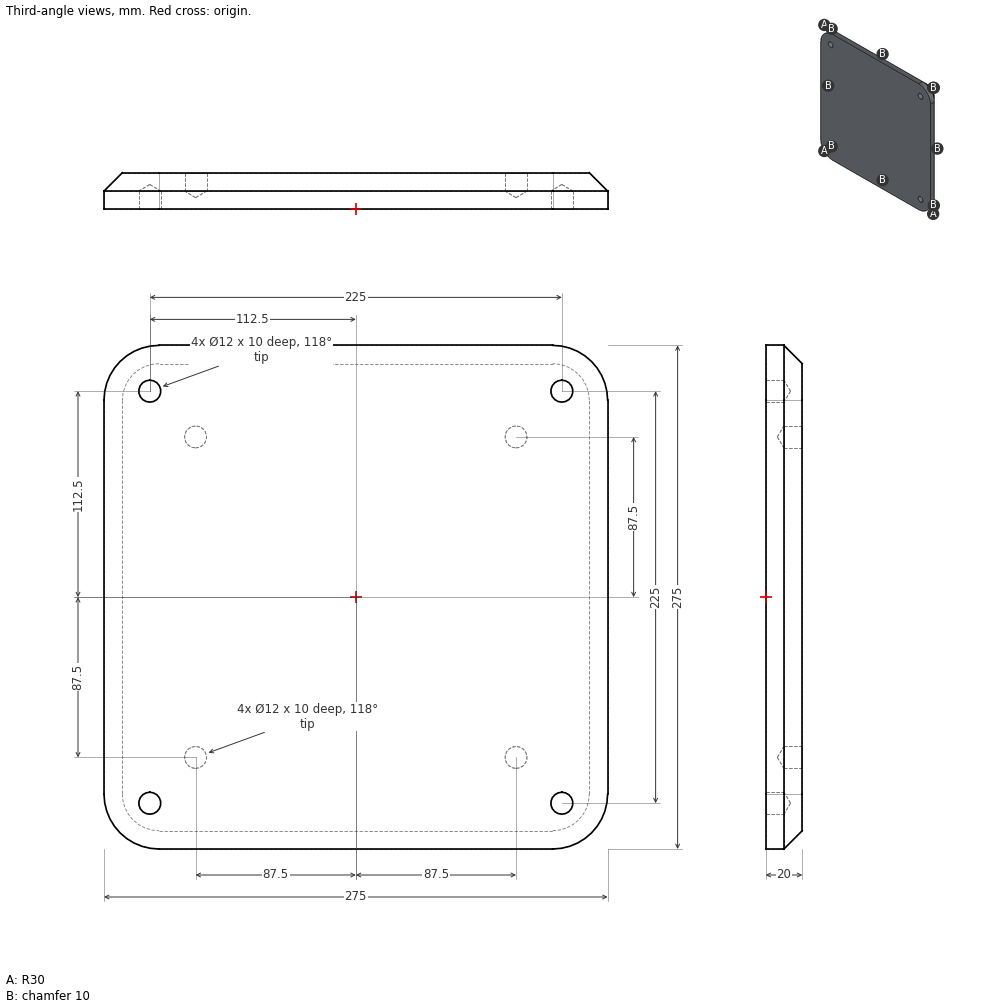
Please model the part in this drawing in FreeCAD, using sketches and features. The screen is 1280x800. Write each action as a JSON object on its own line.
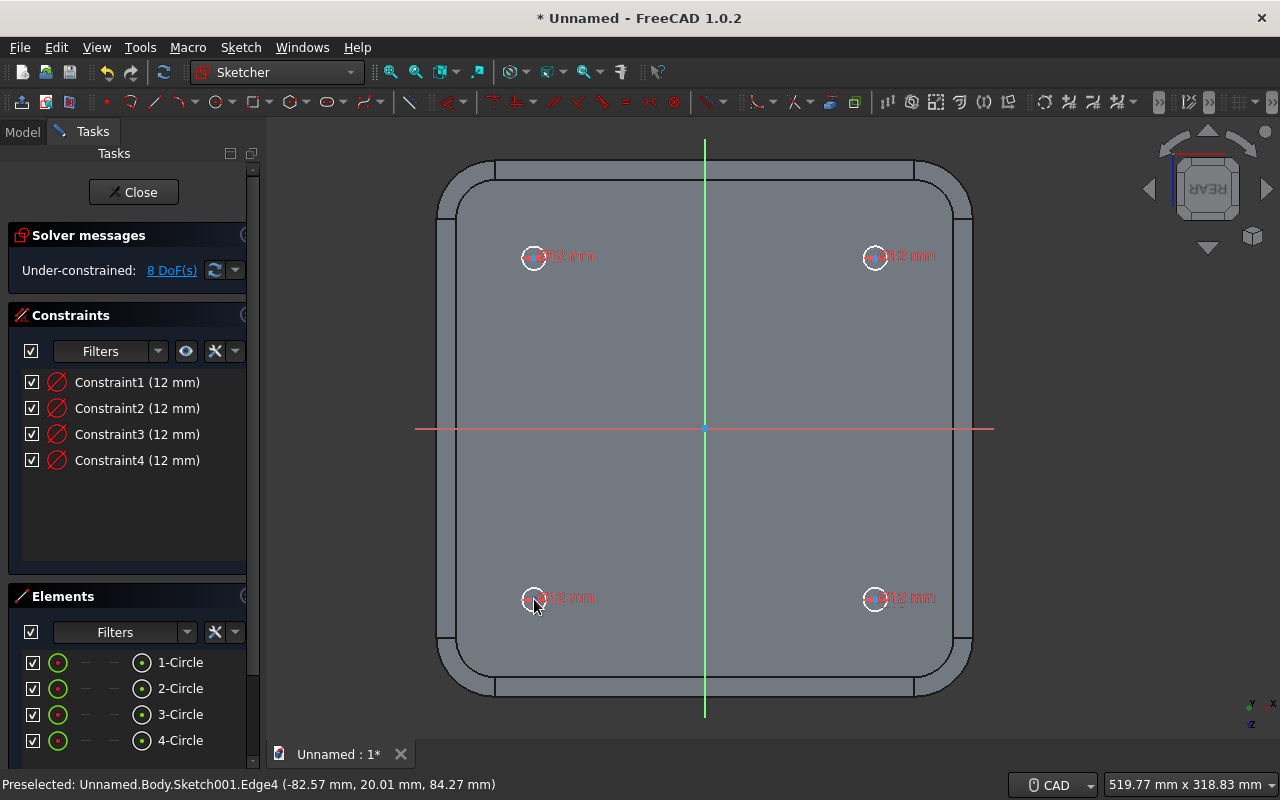
{"action": "left_click", "coordinate": [534, 258]}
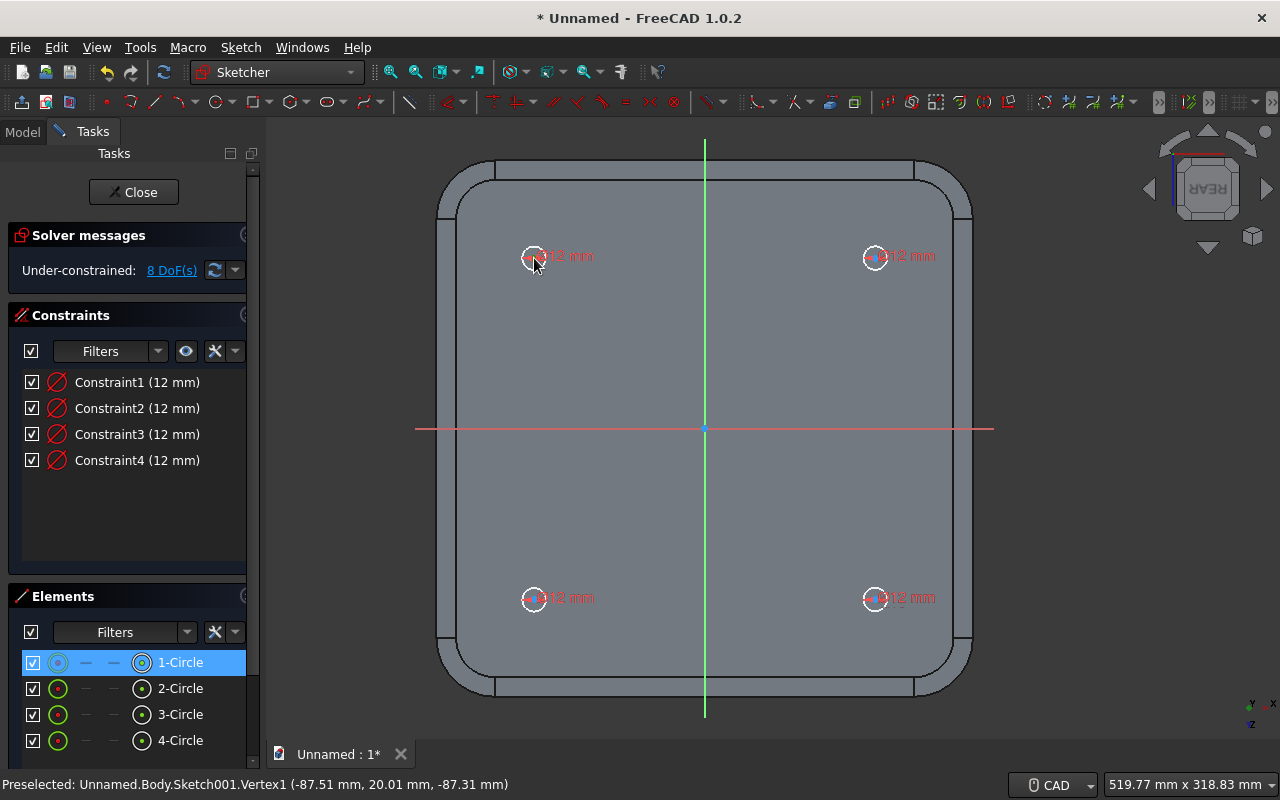
{"action": "left_click", "coordinate": [875, 258]}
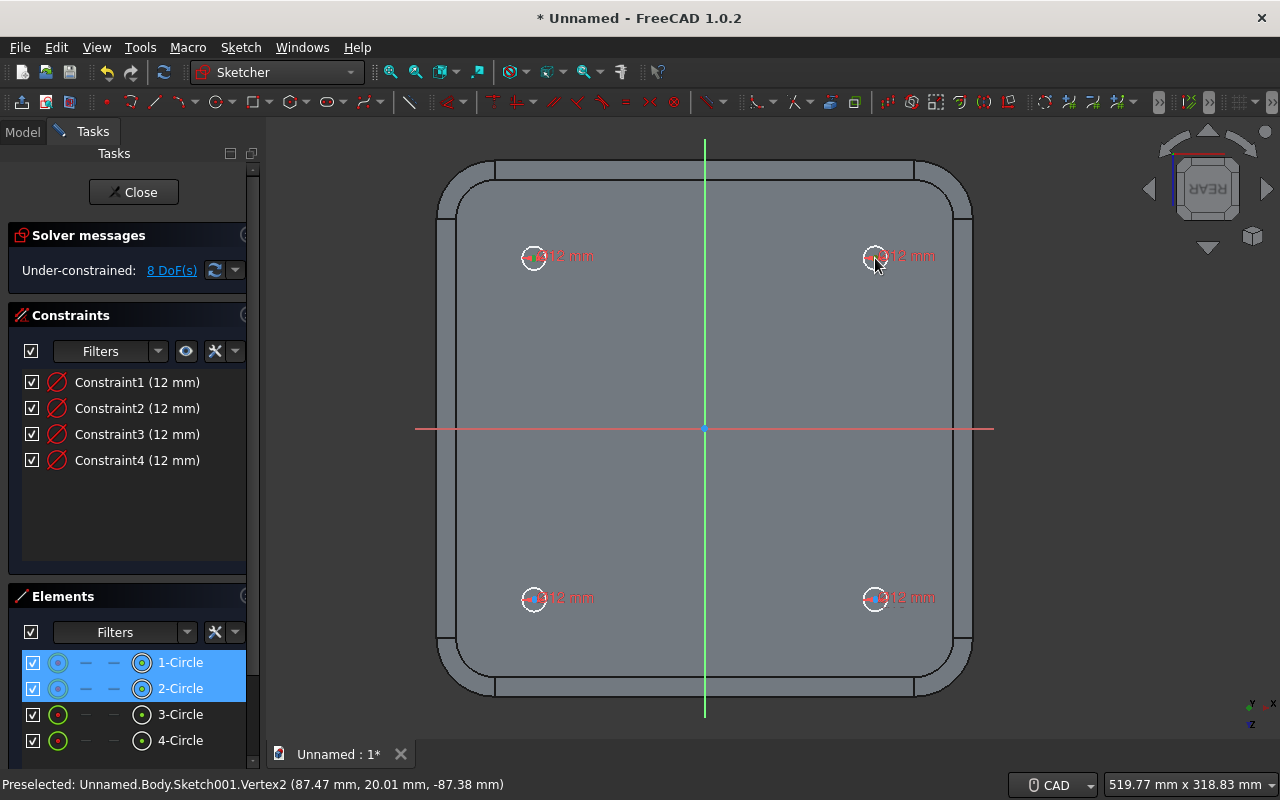
{"action": "key", "text": "h"}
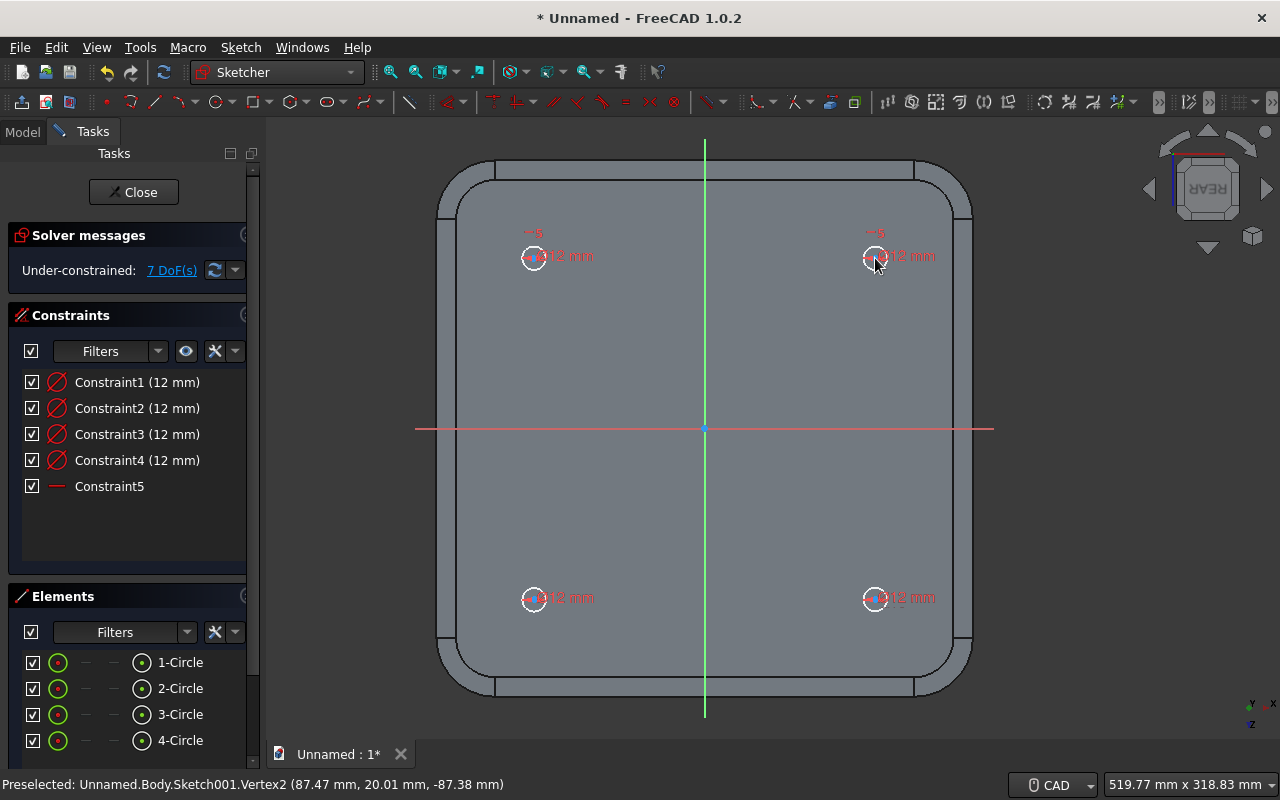
{"action": "left_click", "coordinate": [875, 258]}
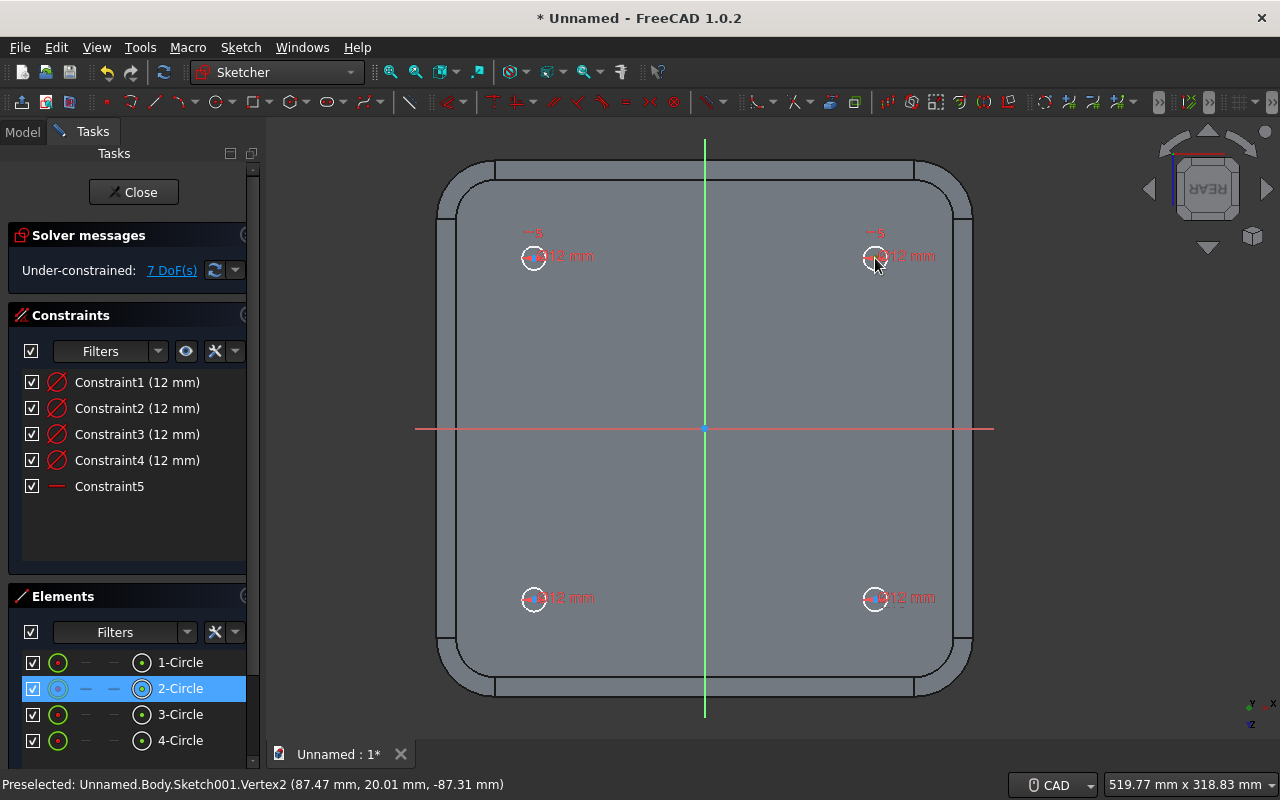
{"action": "left_click", "coordinate": [875, 600]}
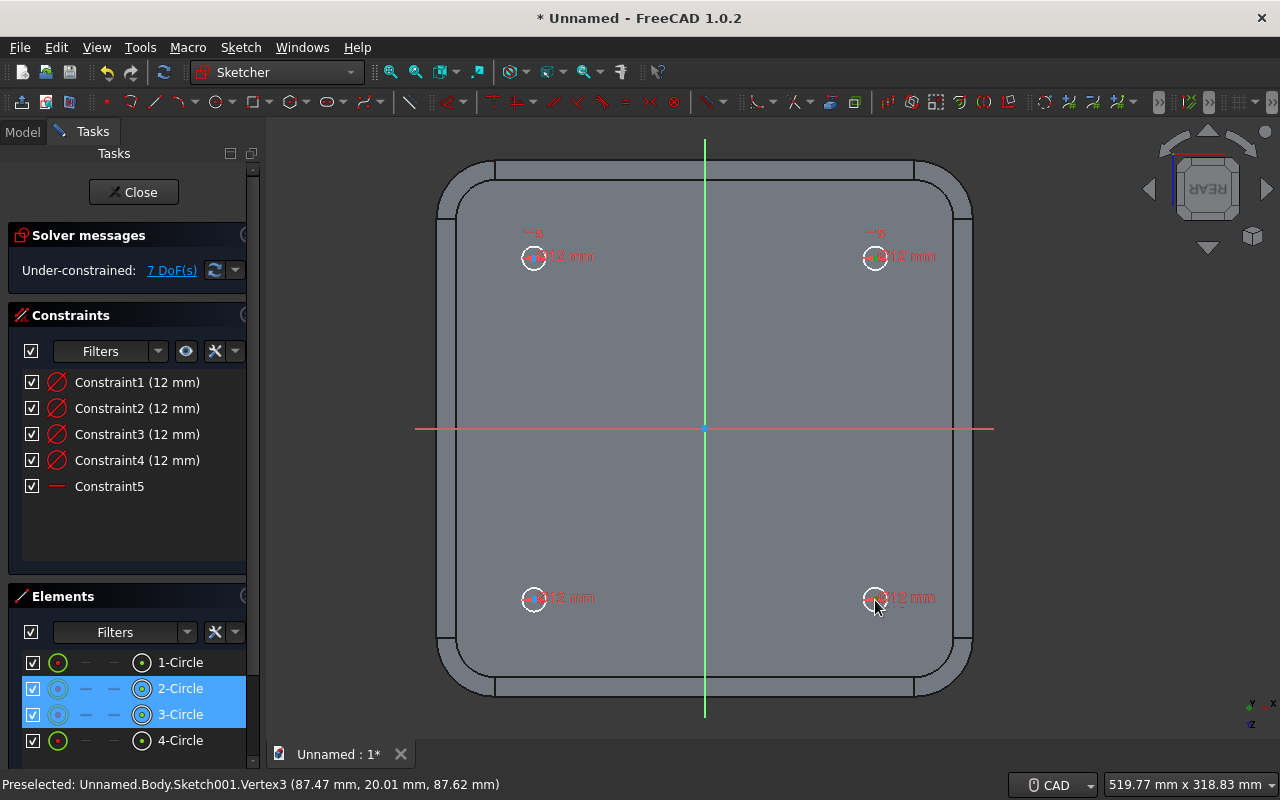
{"action": "key", "text": "v"}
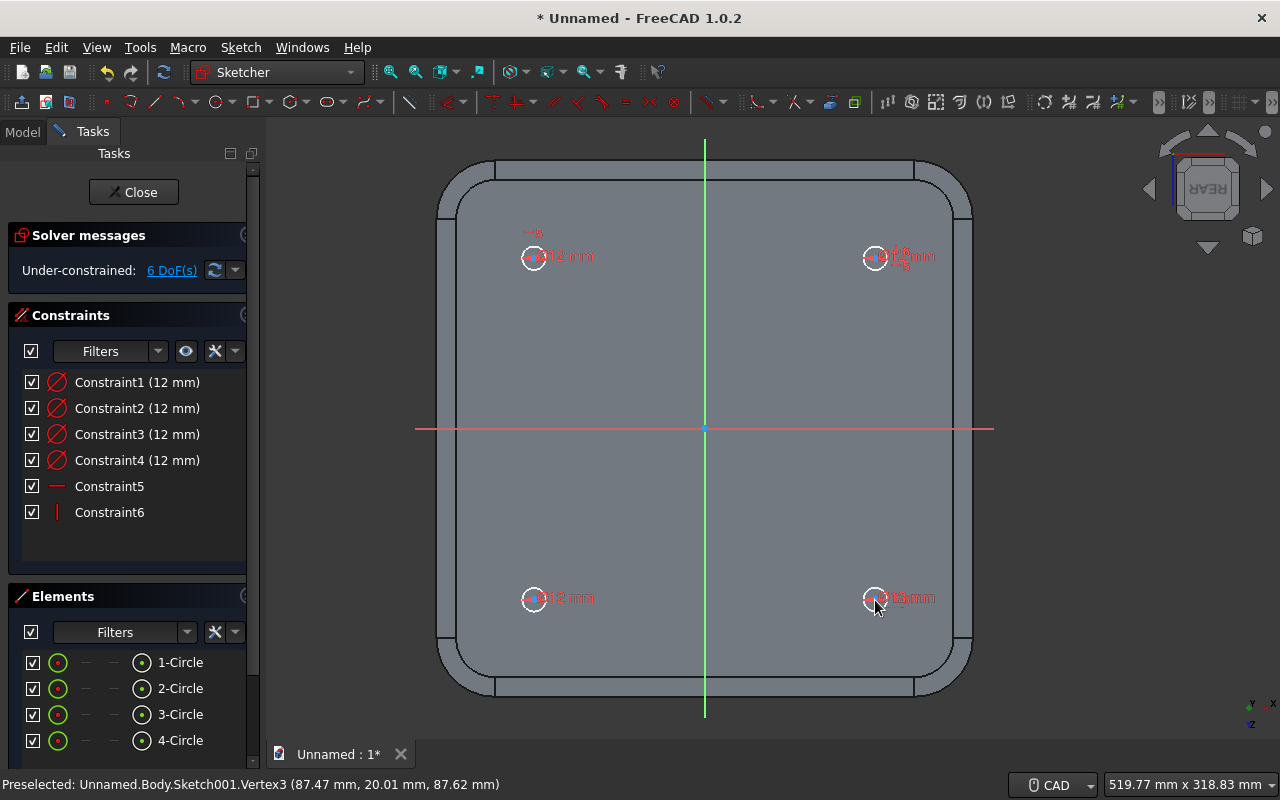
{"action": "left_click", "coordinate": [534, 258]}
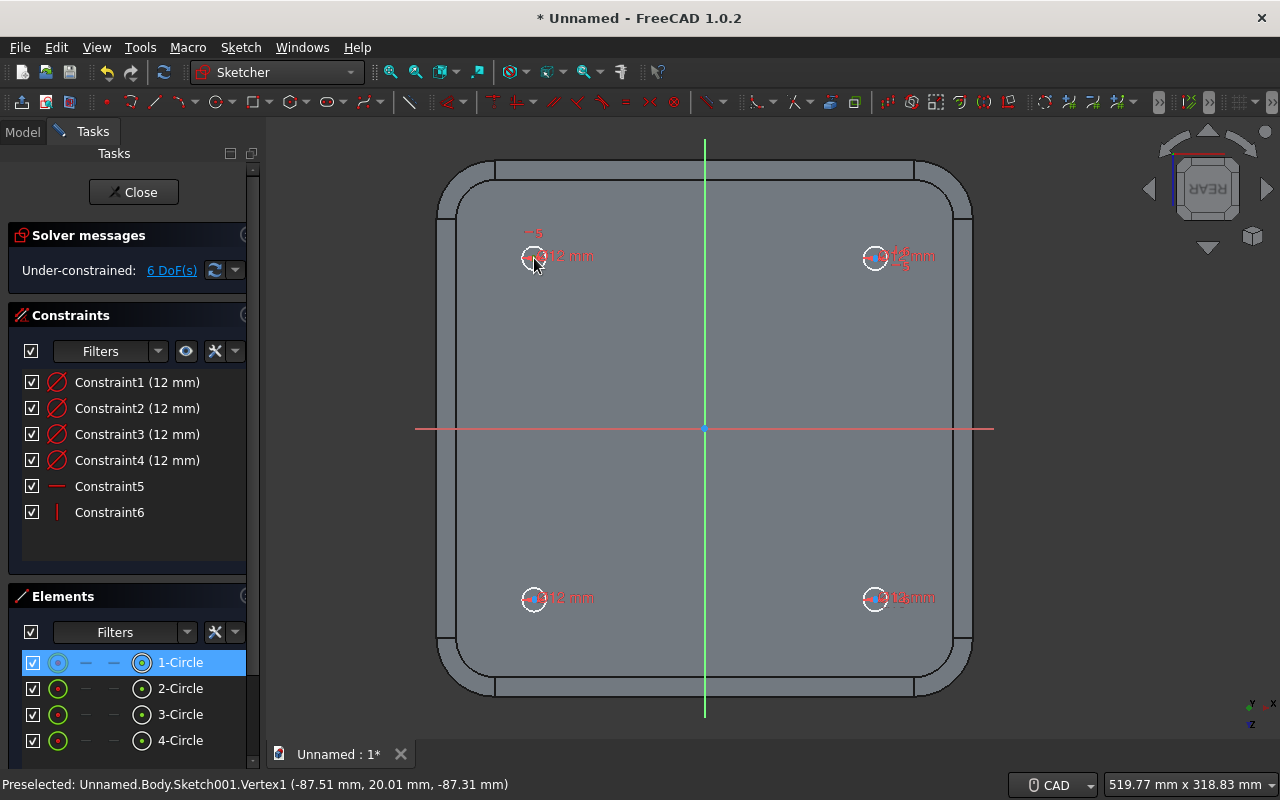
{"action": "left_click", "coordinate": [534, 600]}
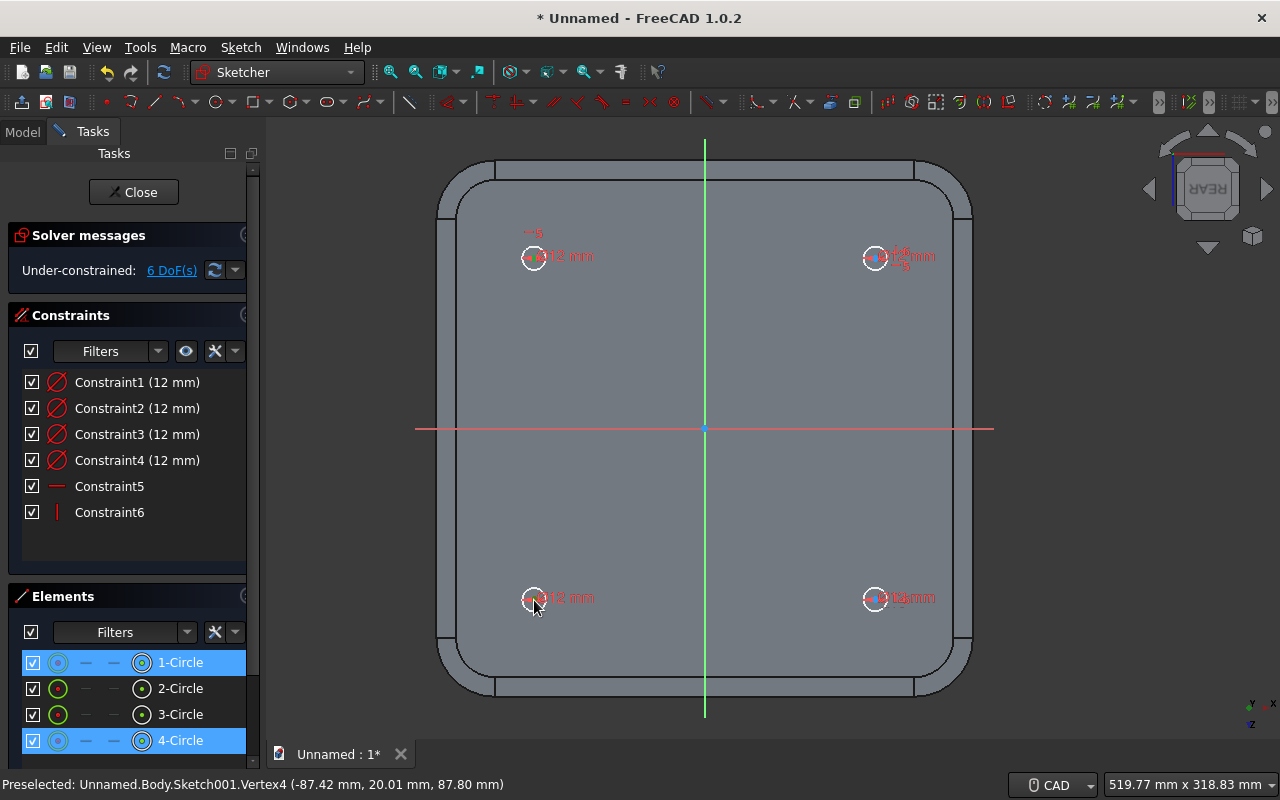
{"action": "left_click", "coordinate": [536, 102]}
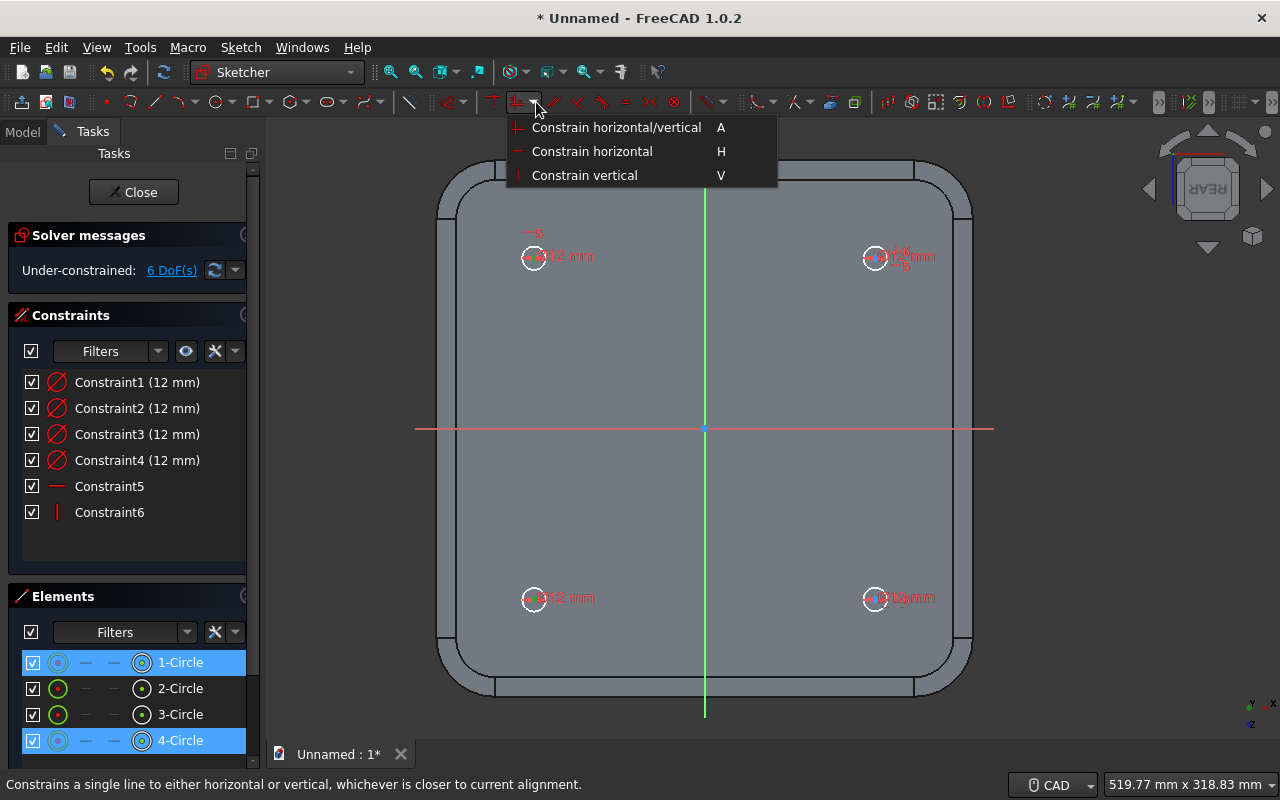
{"action": "left_click", "coordinate": [642, 175]}